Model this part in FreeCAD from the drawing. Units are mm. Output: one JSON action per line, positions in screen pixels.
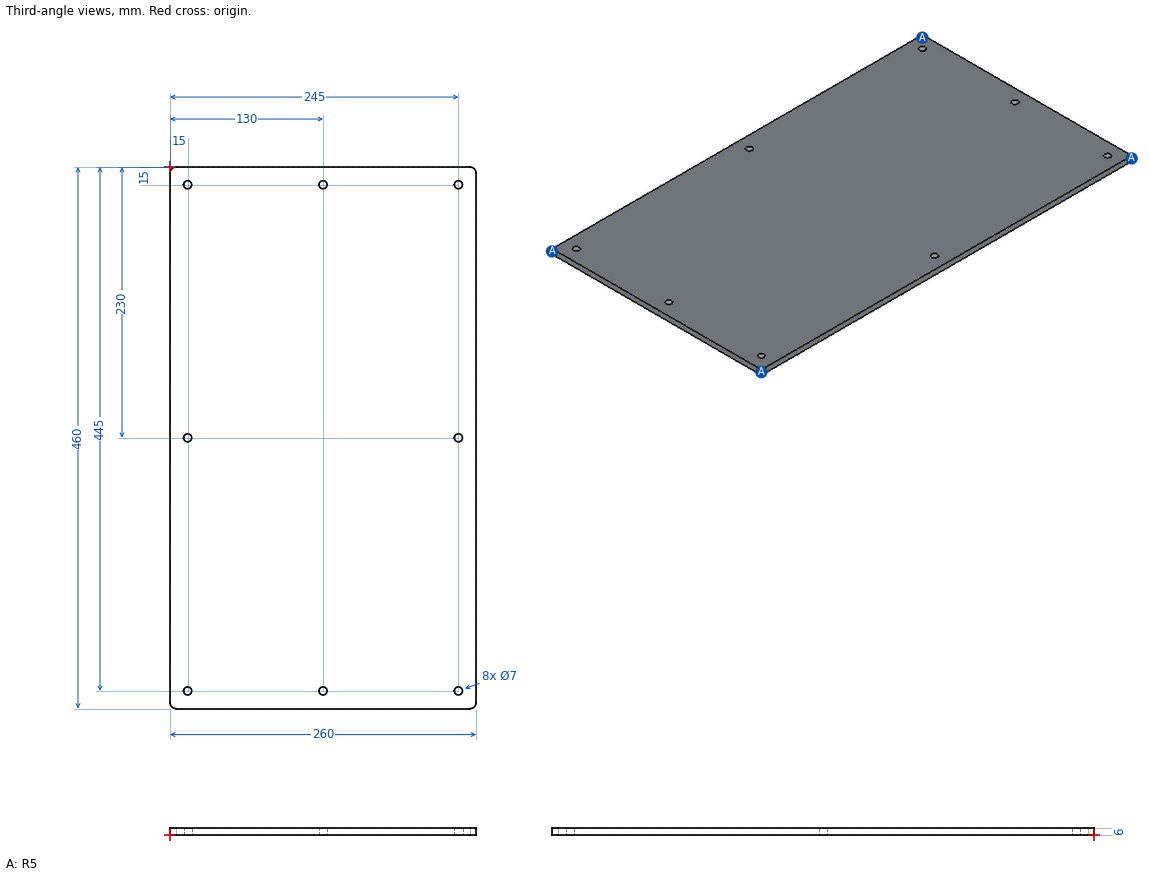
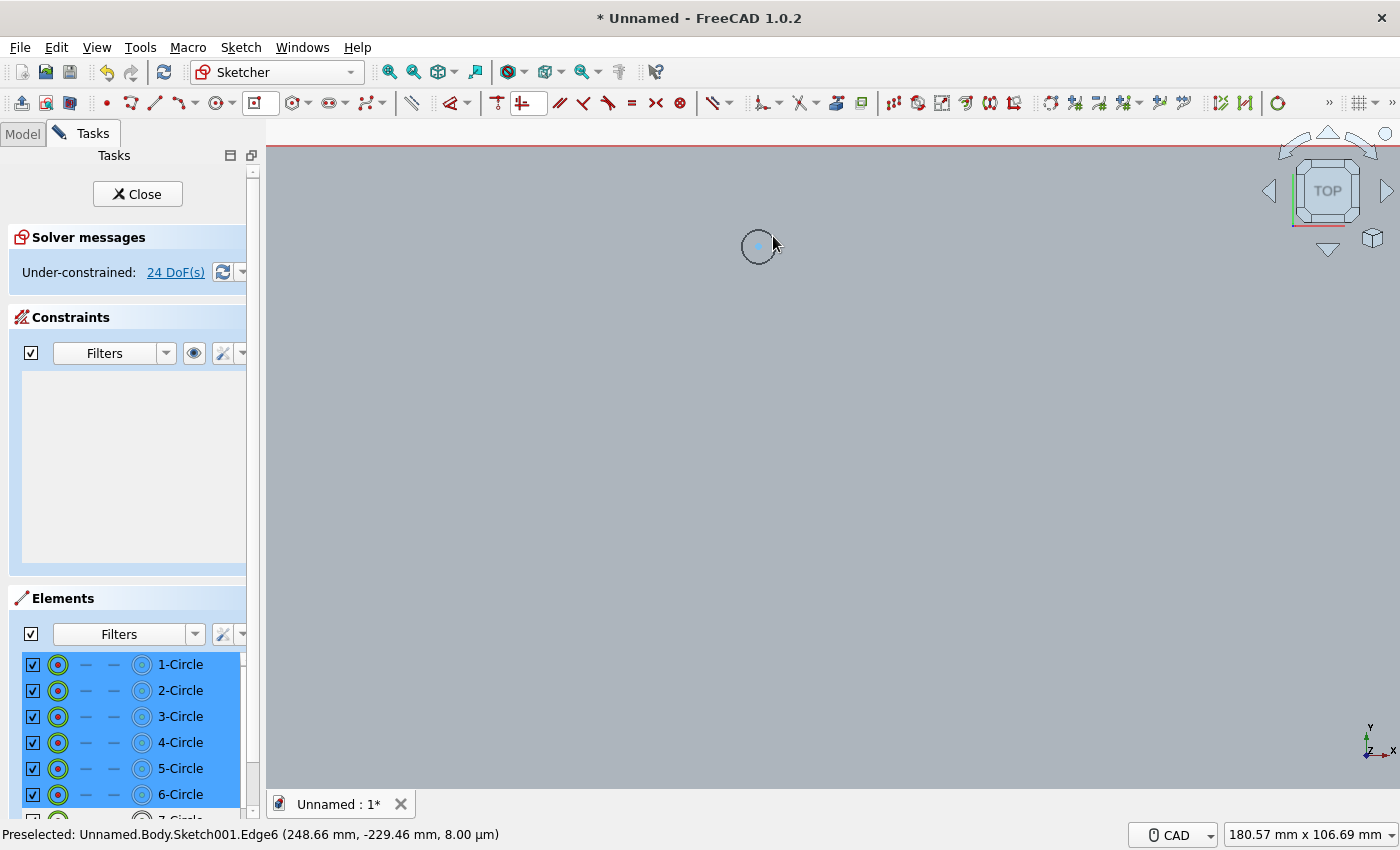
{"action": "left_click", "coordinate": [770, 235]}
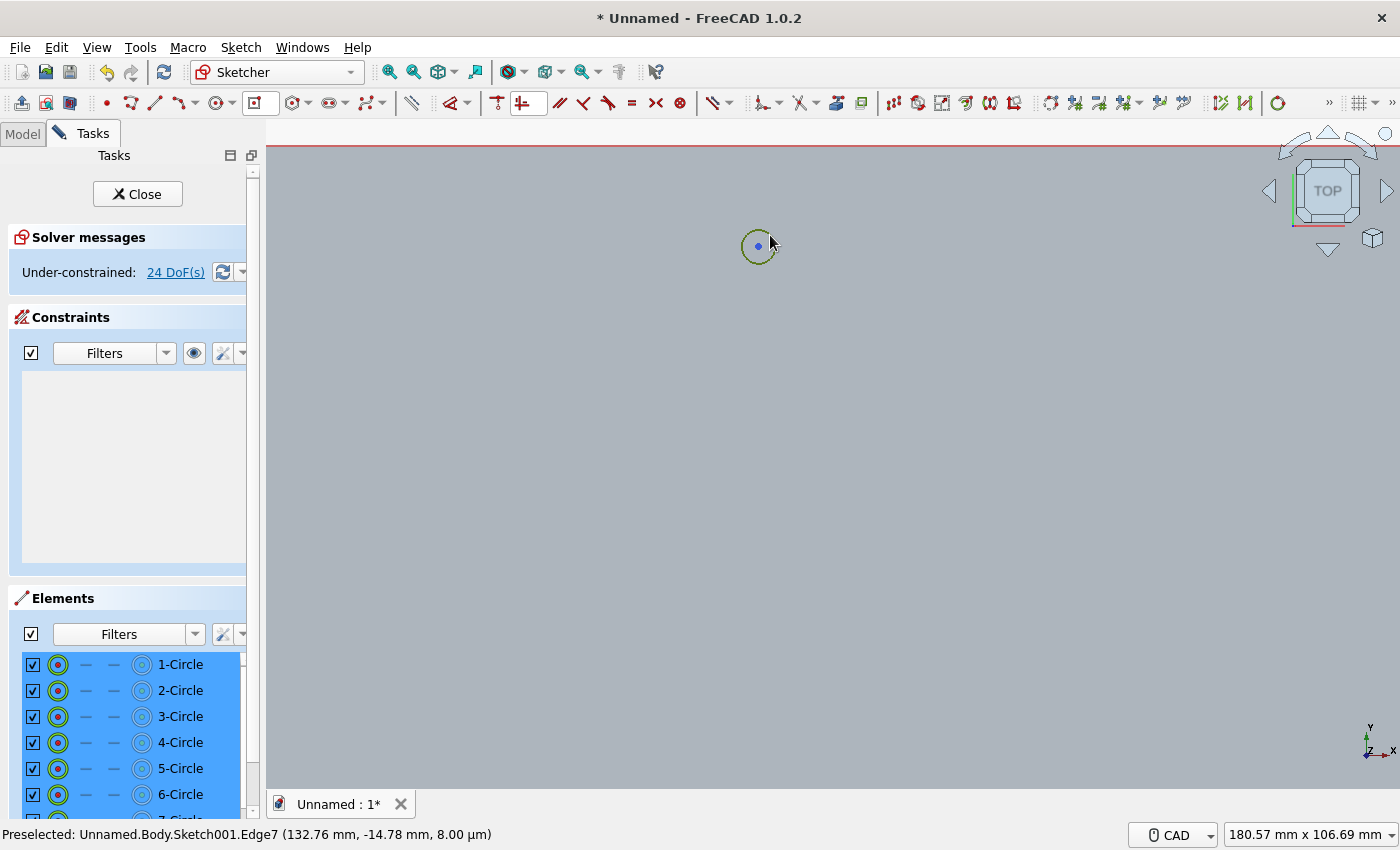
{"action": "scroll", "coordinate": [773, 236], "scroll_direction": "down", "scroll_amount": 9}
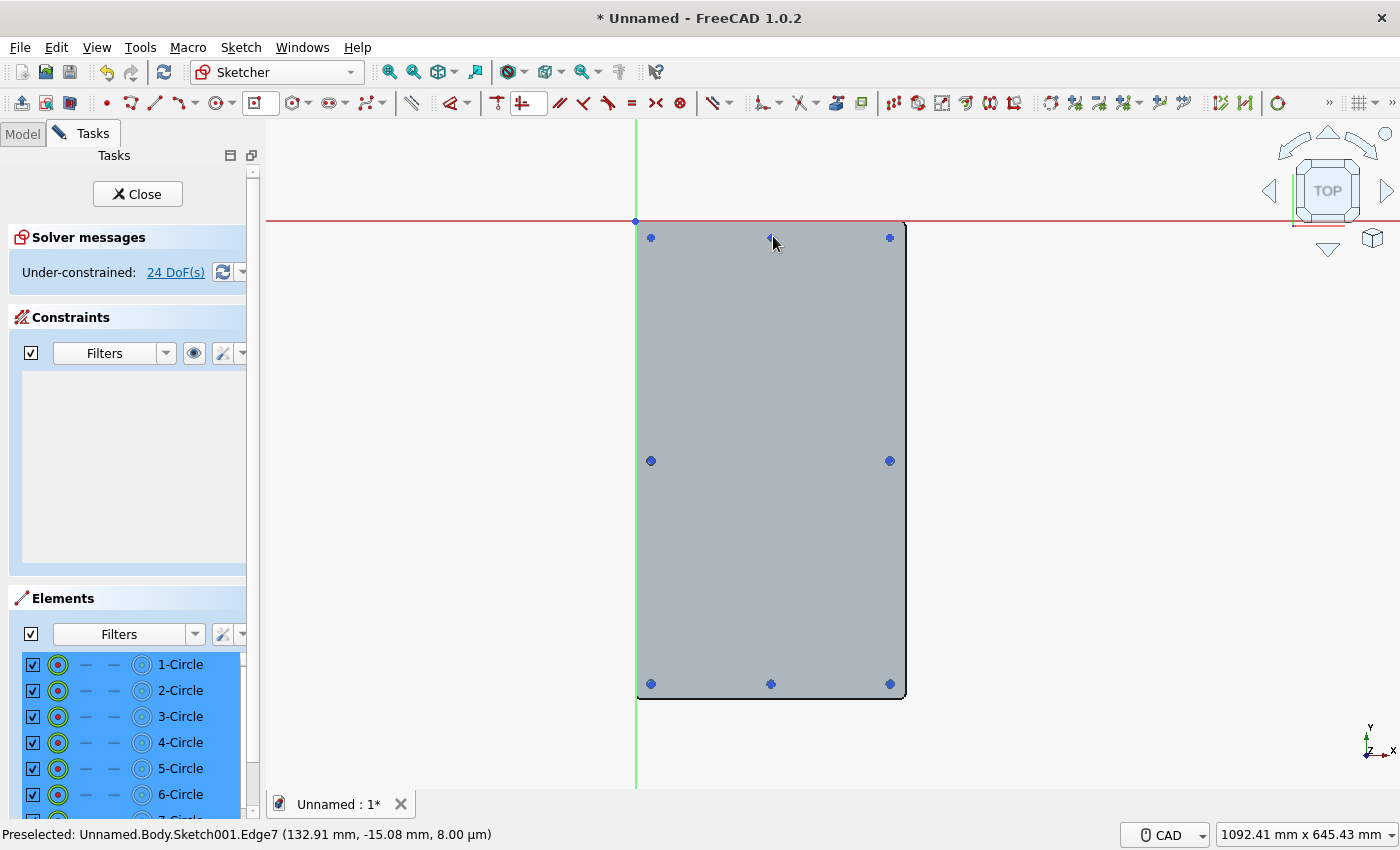
{"action": "scroll", "coordinate": [654, 458], "scroll_direction": "up", "scroll_amount": 6}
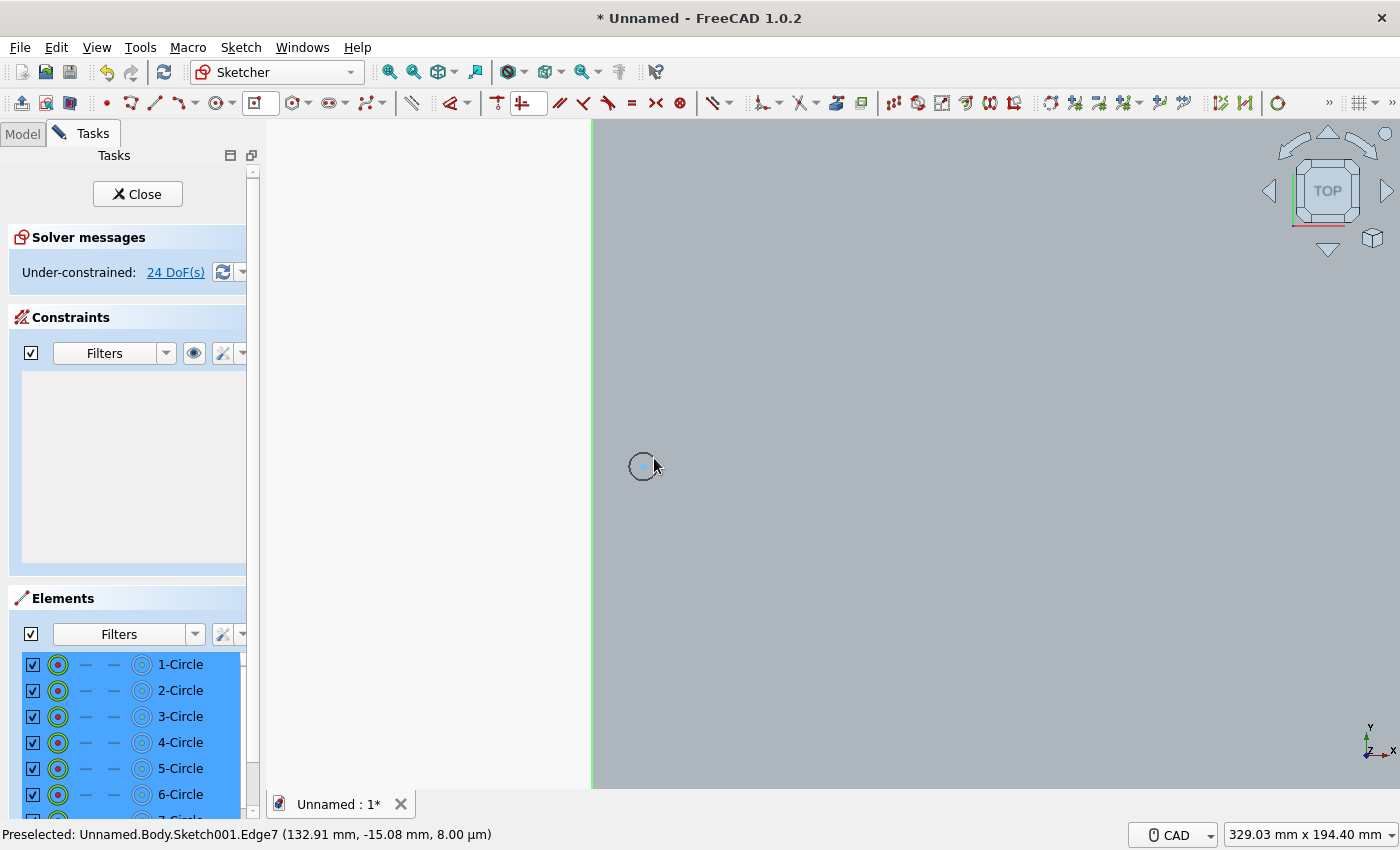
{"action": "left_click", "coordinate": [653, 457]}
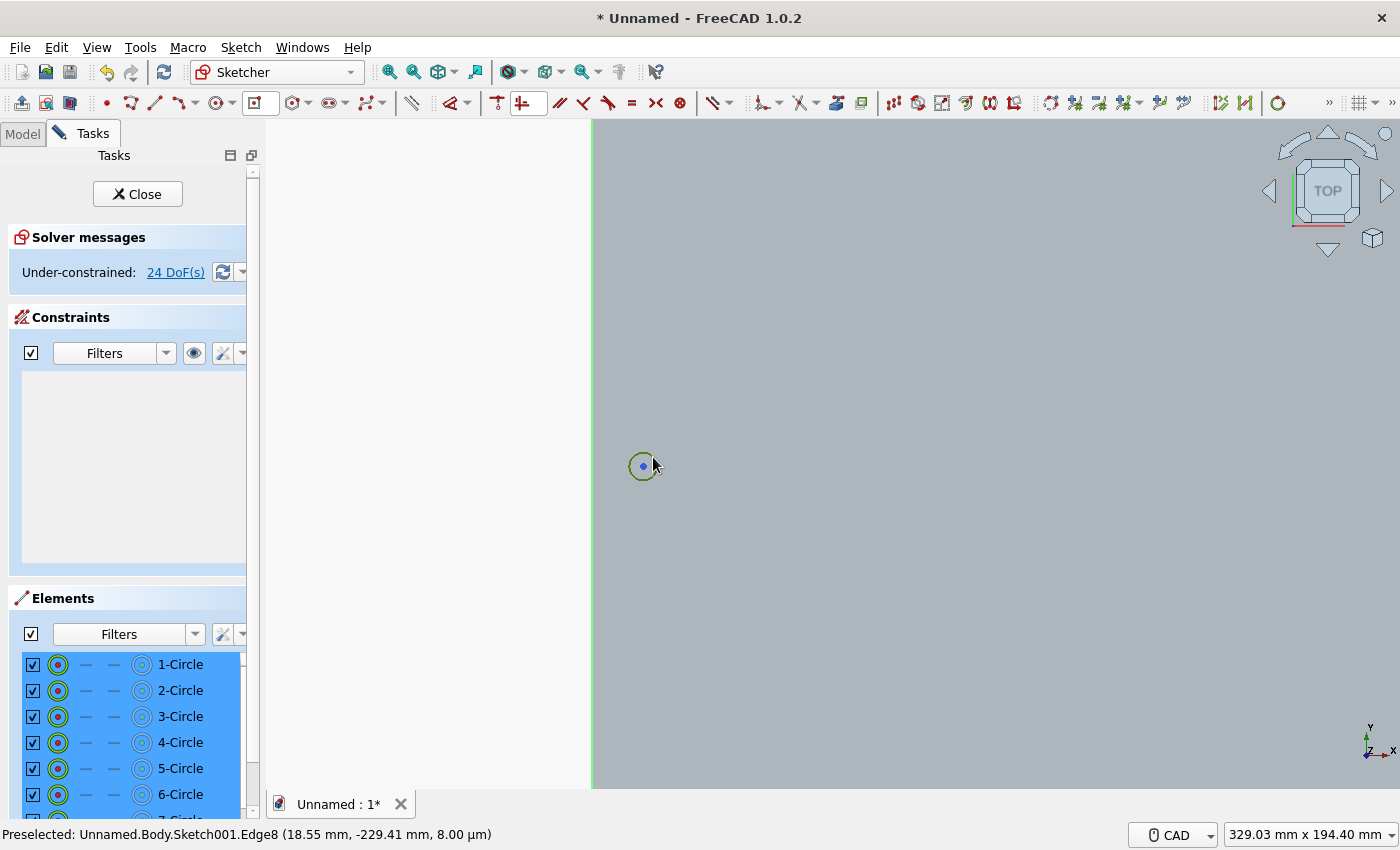
{"action": "key", "text": "e"}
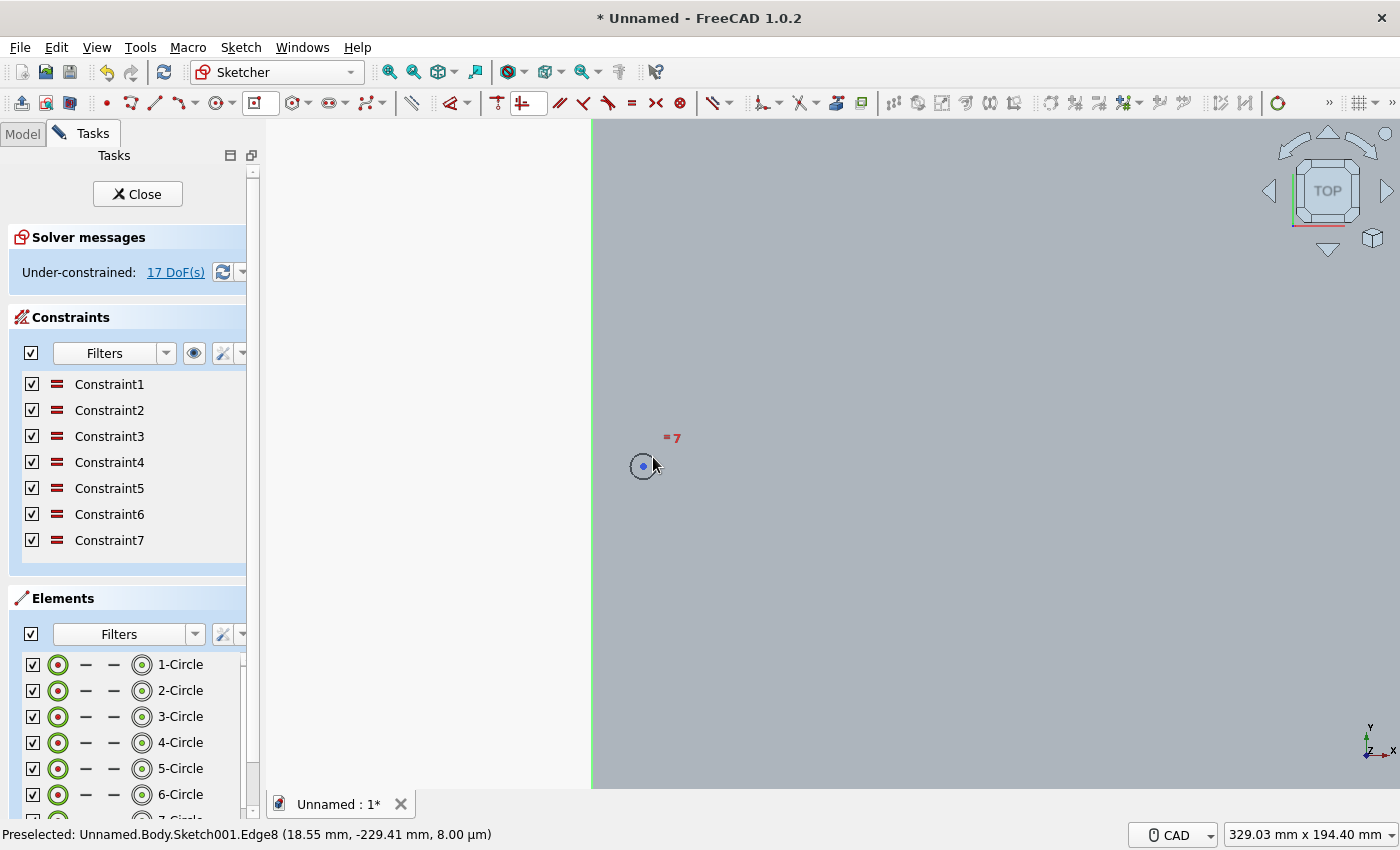
{"action": "scroll", "coordinate": [654, 458], "scroll_direction": "down", "scroll_amount": 6}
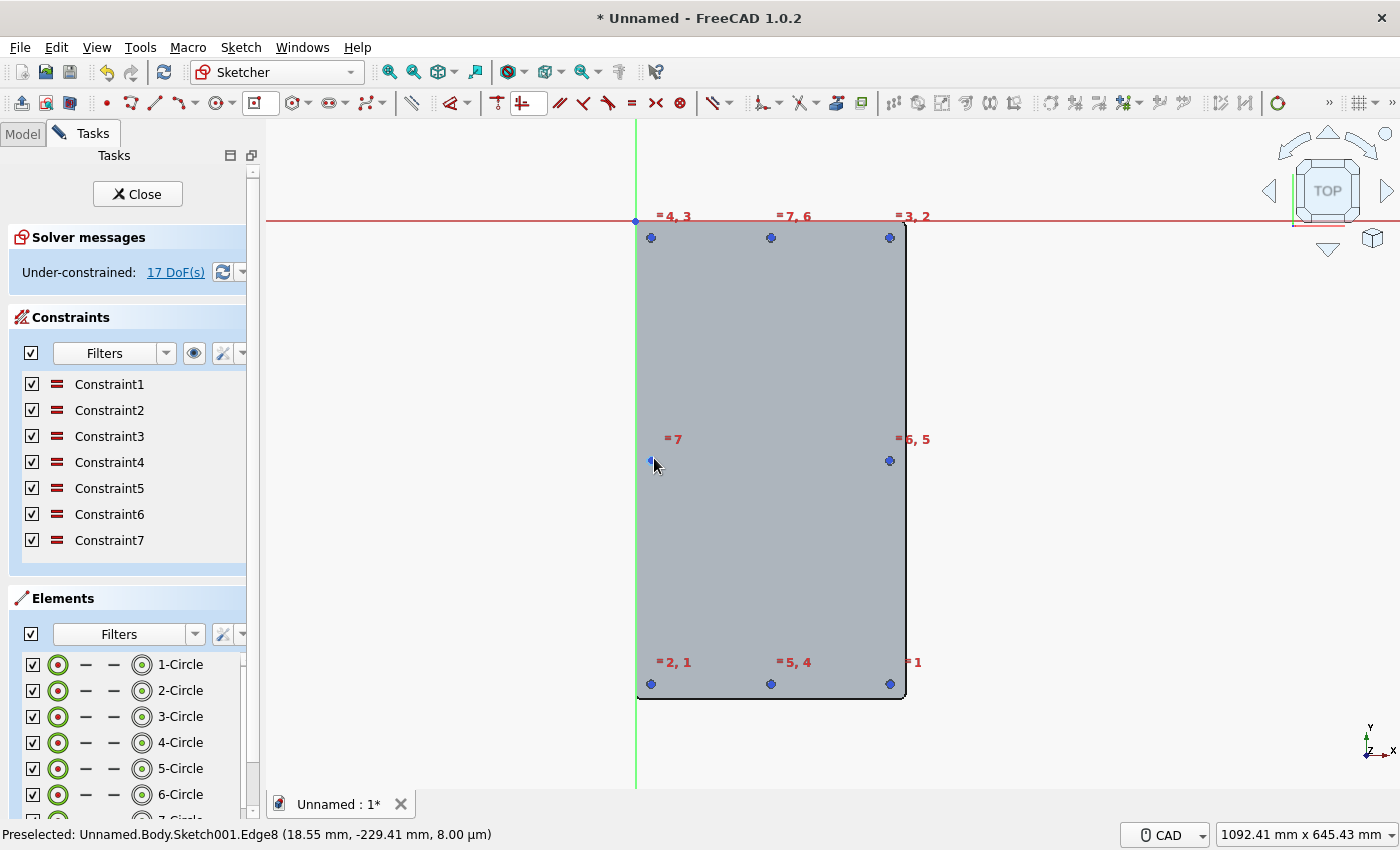
{"action": "scroll", "coordinate": [893, 681], "scroll_direction": "up", "scroll_amount": 9}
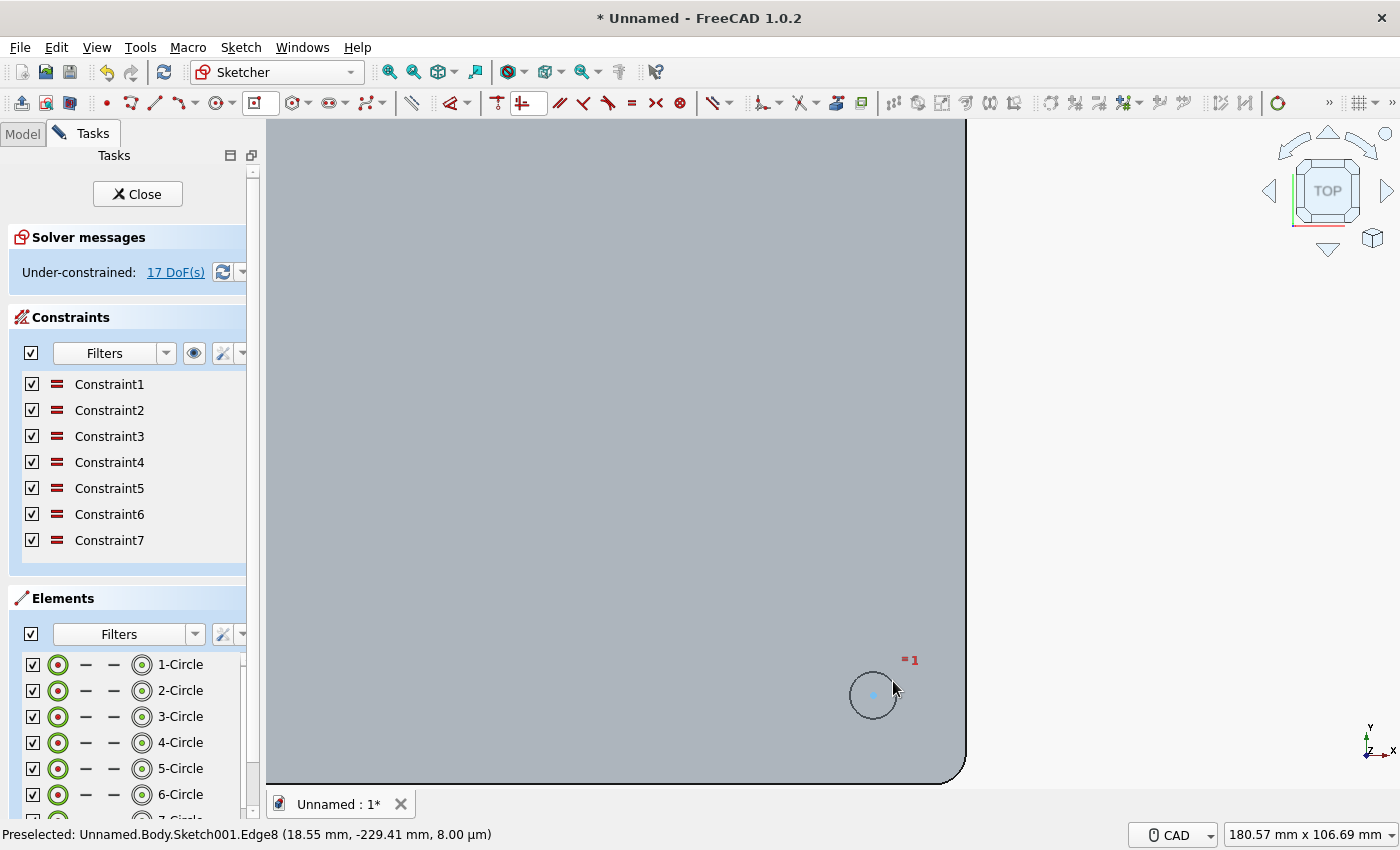
{"action": "left_click", "coordinate": [890, 679]}